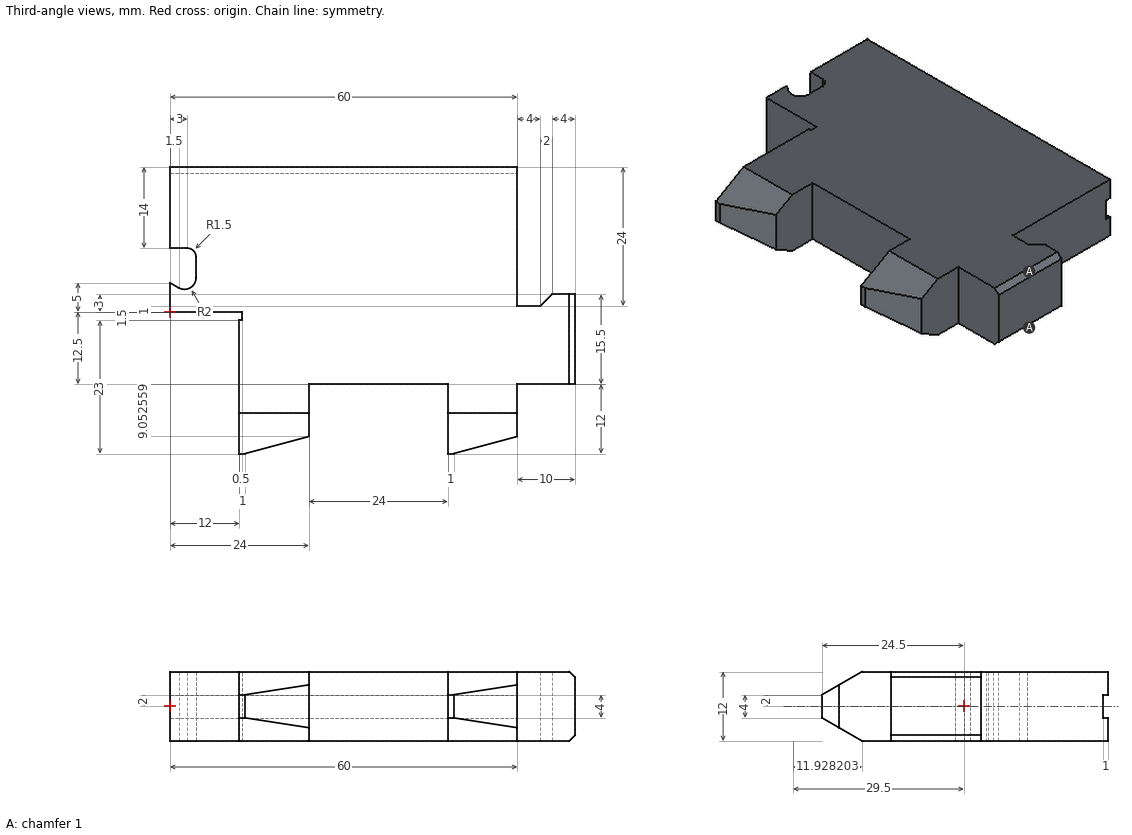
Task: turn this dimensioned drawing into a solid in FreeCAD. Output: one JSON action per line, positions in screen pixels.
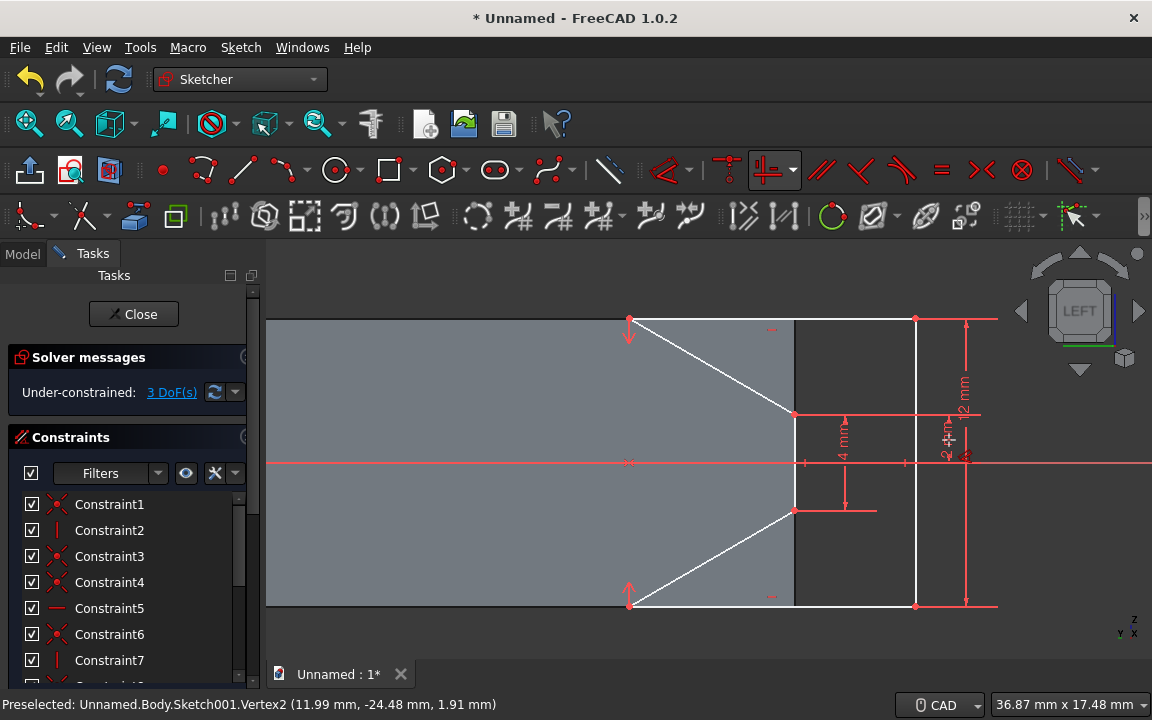
{"action": "left_click", "coordinate": [795, 415]}
{"action": "left_click", "coordinate": [544, 381]}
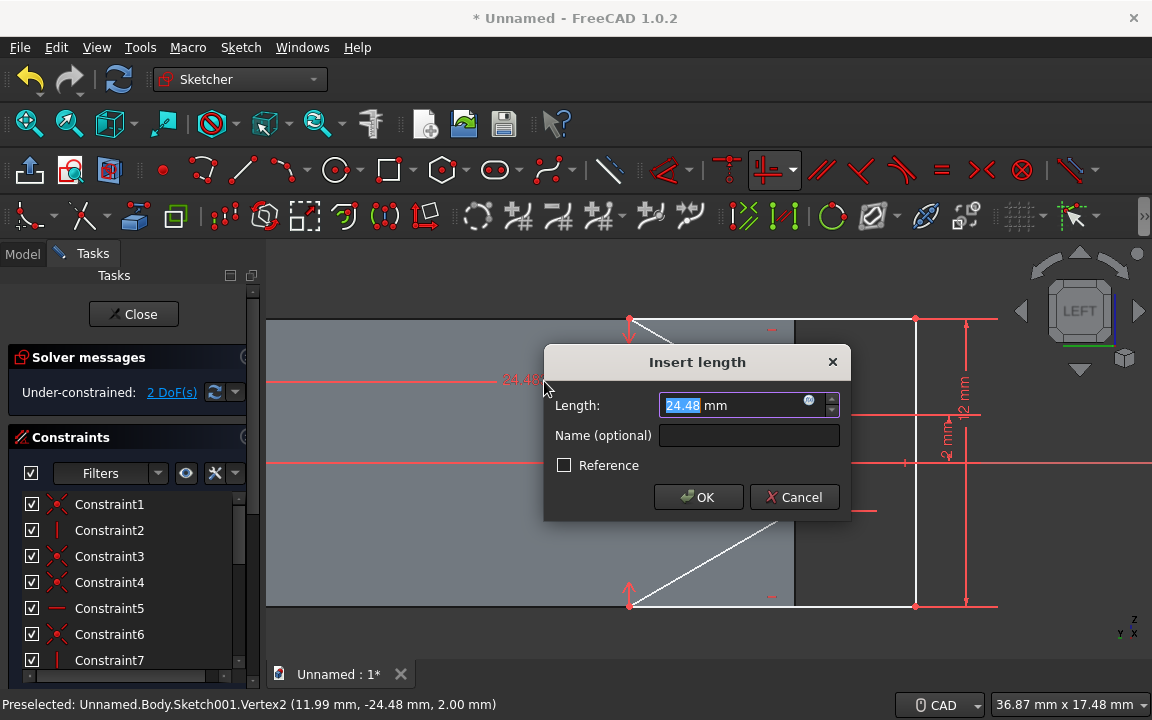
{"action": "type", "text": "24.5"}
{"action": "key", "text": "Return"}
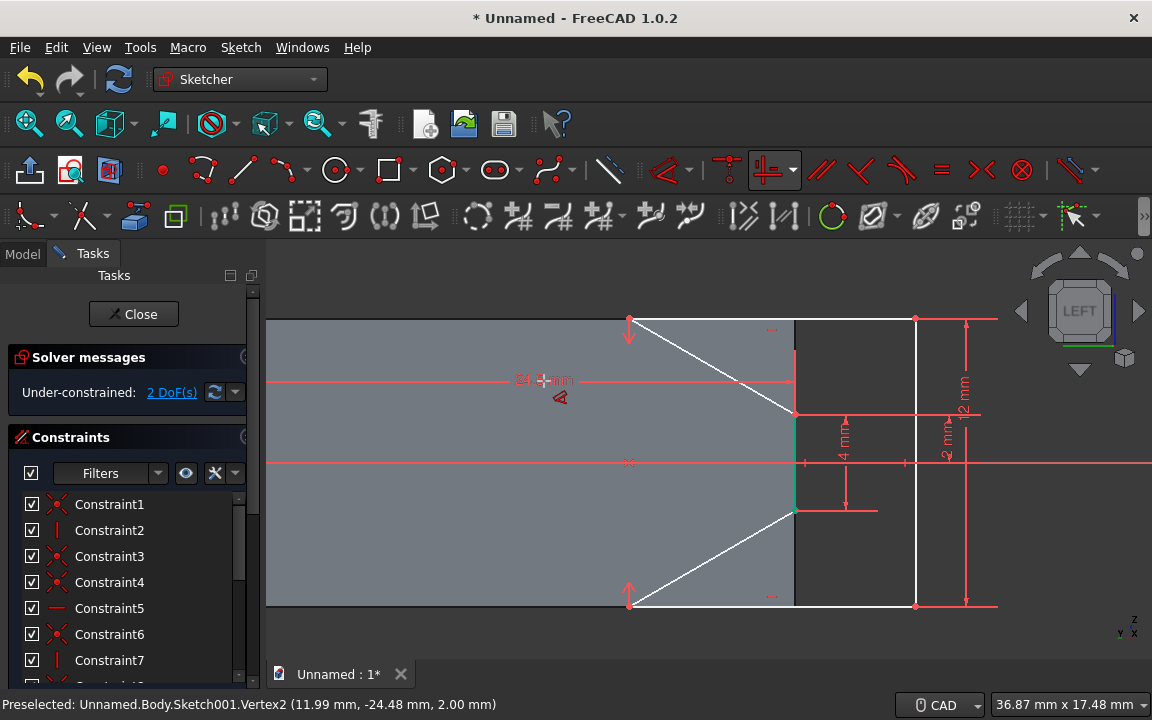
{"action": "left_click", "coordinate": [916, 607]}
{"action": "left_click", "coordinate": [605, 429]}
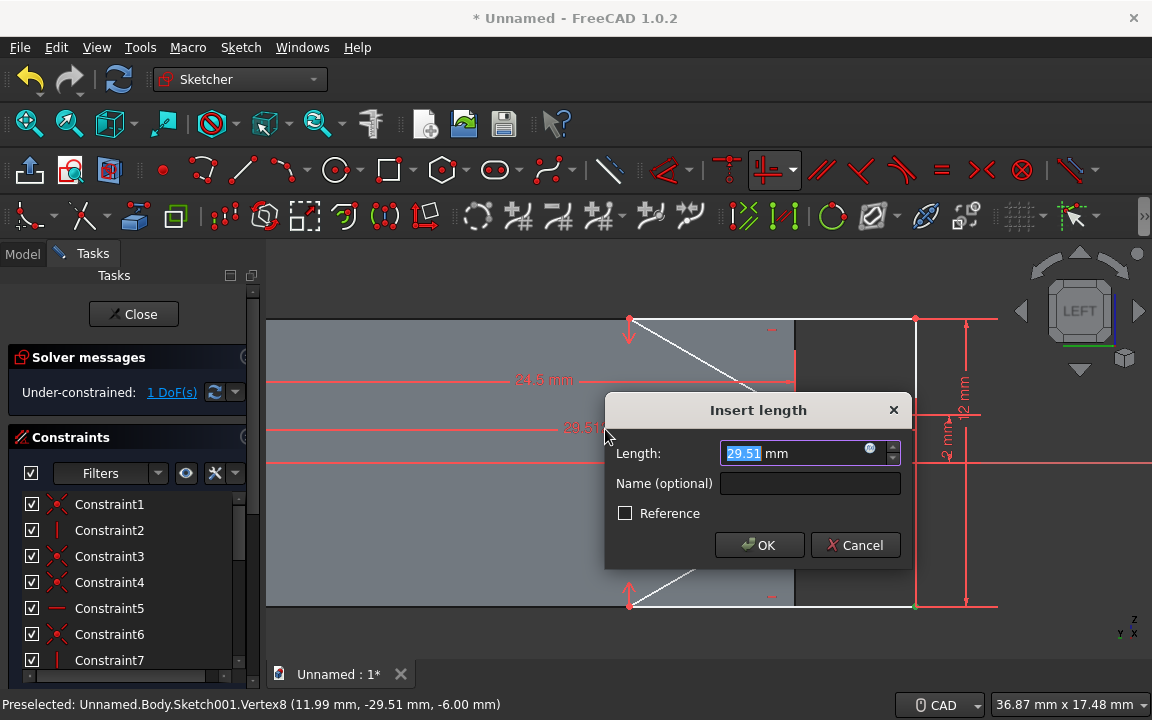
{"action": "type", "text": "29.5"}
{"action": "key", "text": "Return"}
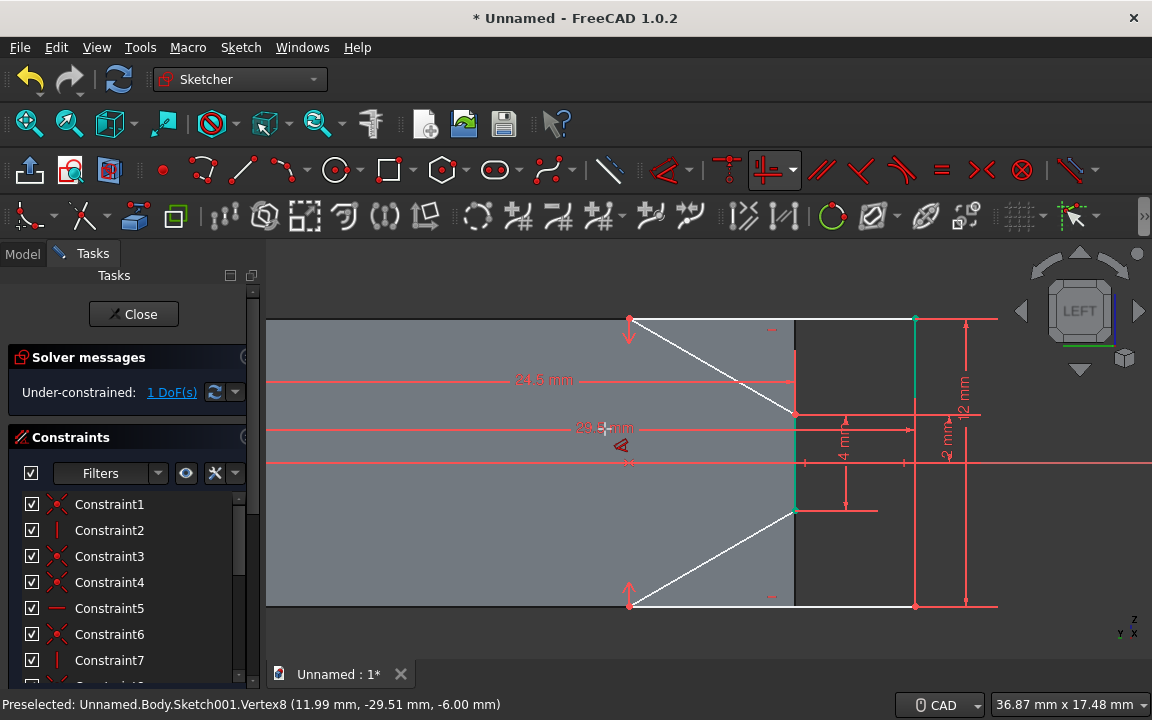
{"action": "left_click", "coordinate": [715, 607]}
{"action": "left_click", "coordinate": [772, 573]}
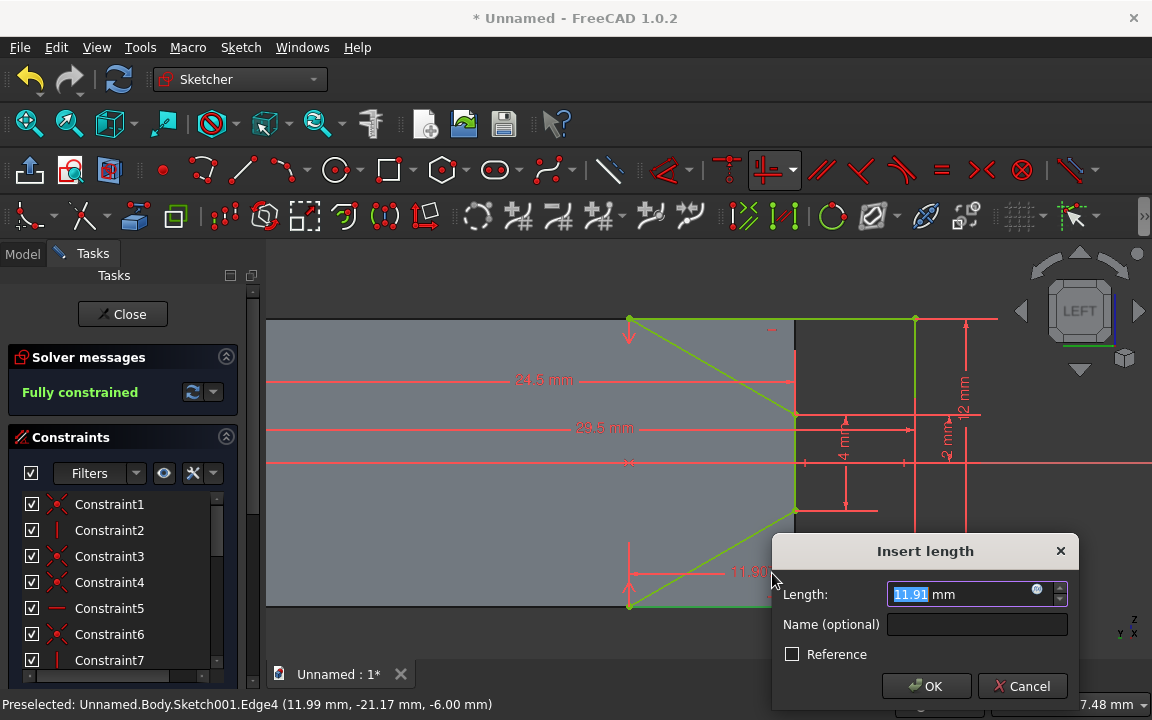
{"action": "type", "text": "11.928203"}
{"action": "key", "text": "Return"}
{"action": "key", "text": "Escape"}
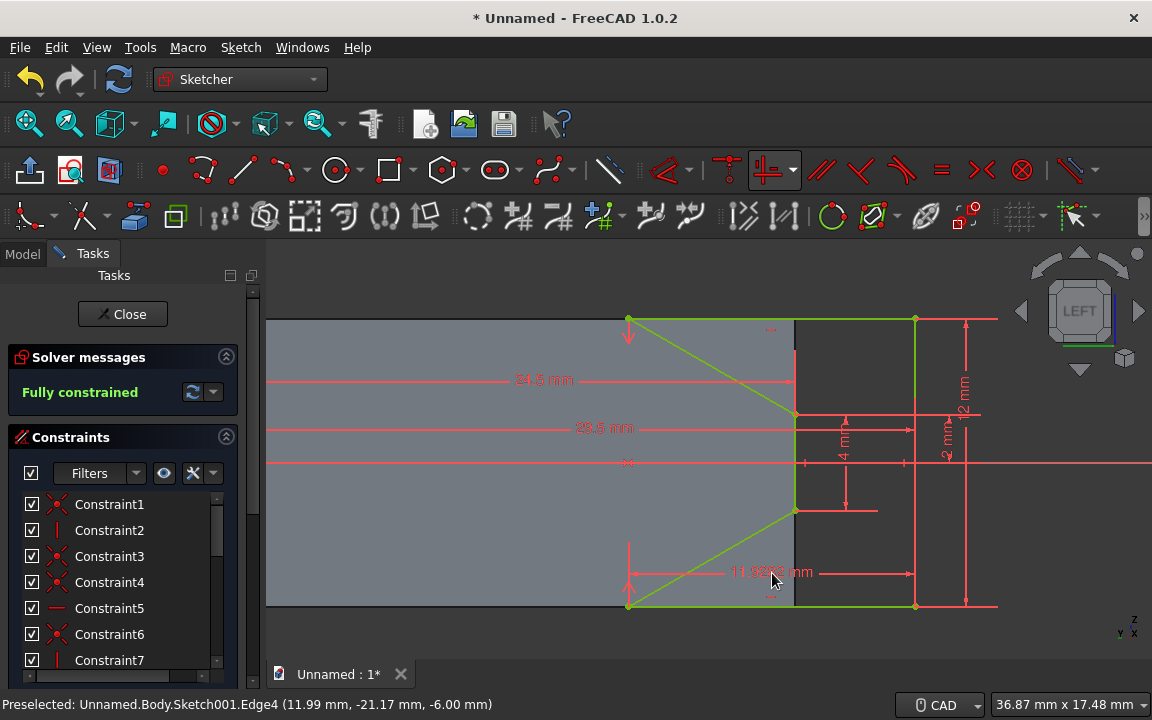
{"action": "left_click", "coordinate": [123, 314]}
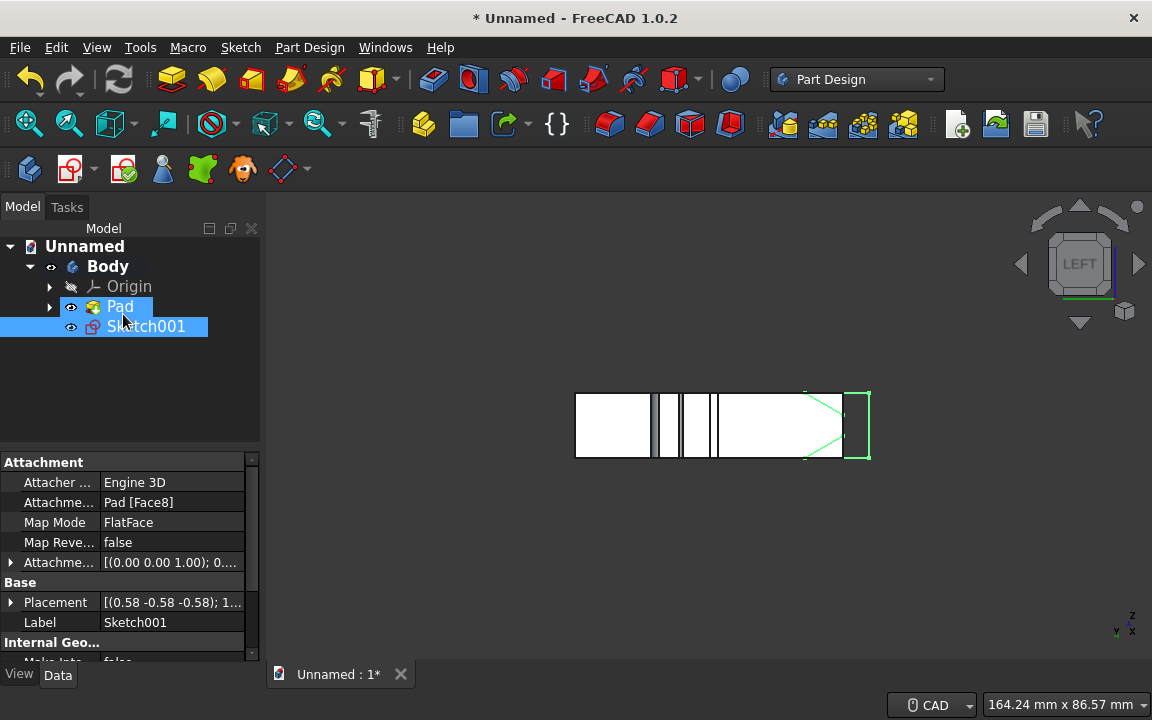
{"action": "left_click", "coordinate": [434, 80]}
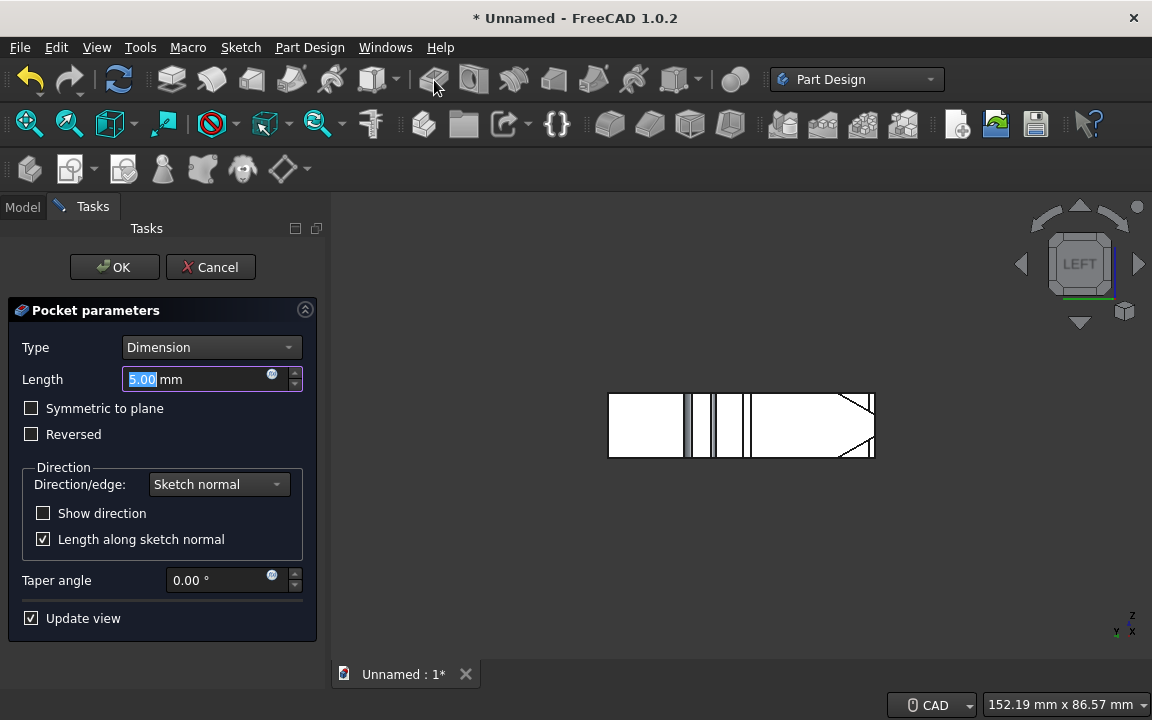
{"action": "left_click", "coordinate": [212, 348]}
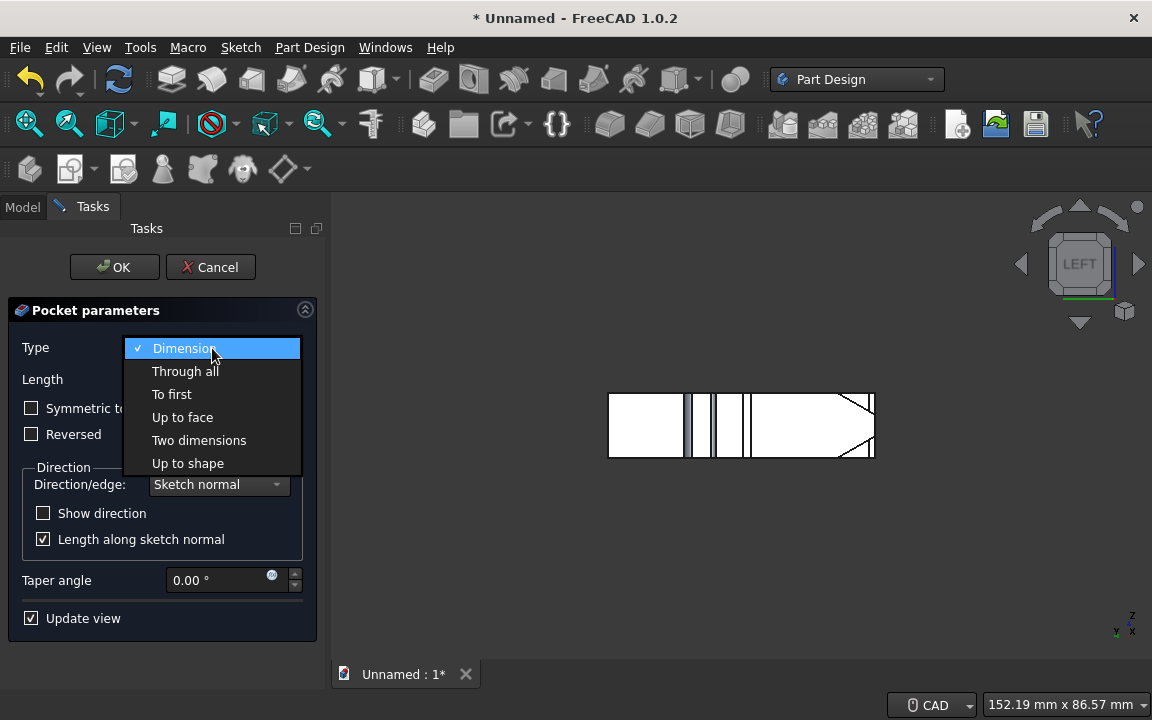
{"action": "left_click", "coordinate": [212, 372]}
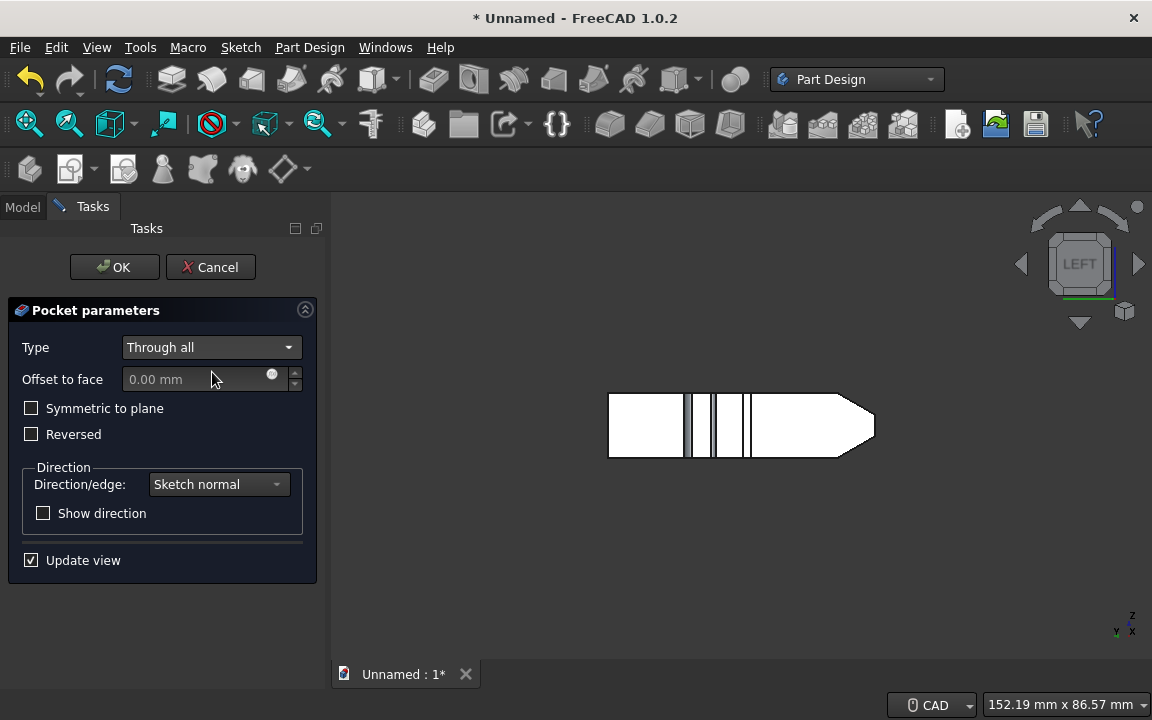
{"action": "left_click", "coordinate": [115, 267]}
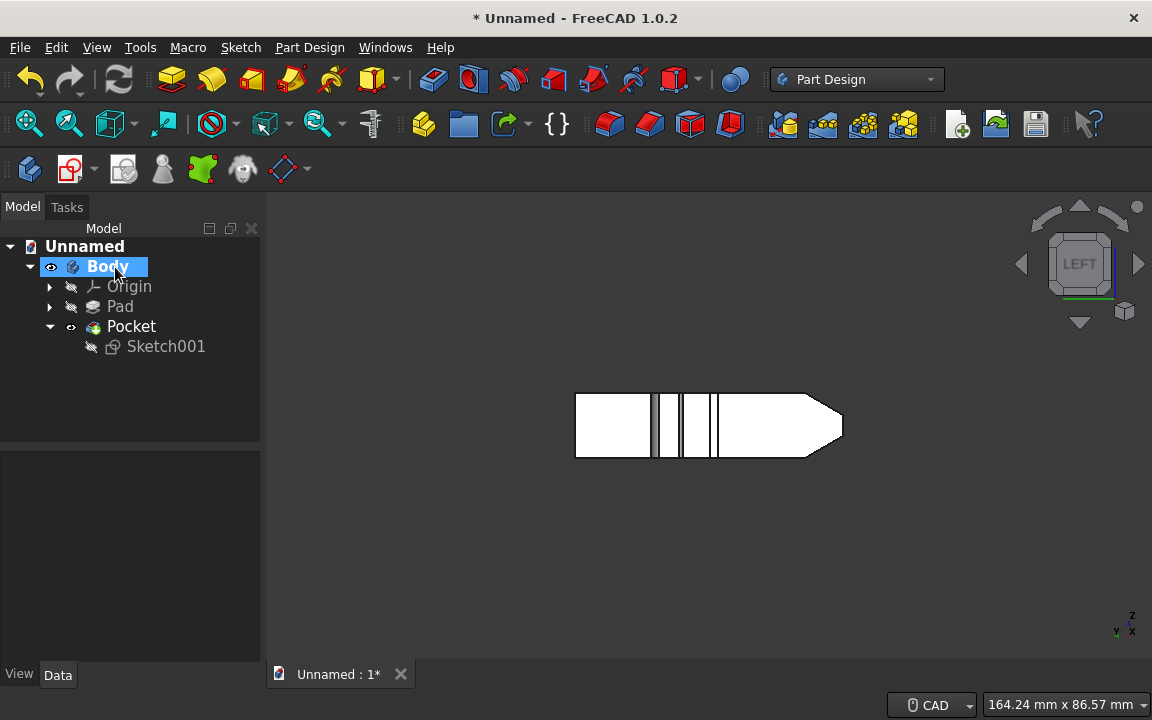
{"action": "left_click", "coordinate": [30, 124]}